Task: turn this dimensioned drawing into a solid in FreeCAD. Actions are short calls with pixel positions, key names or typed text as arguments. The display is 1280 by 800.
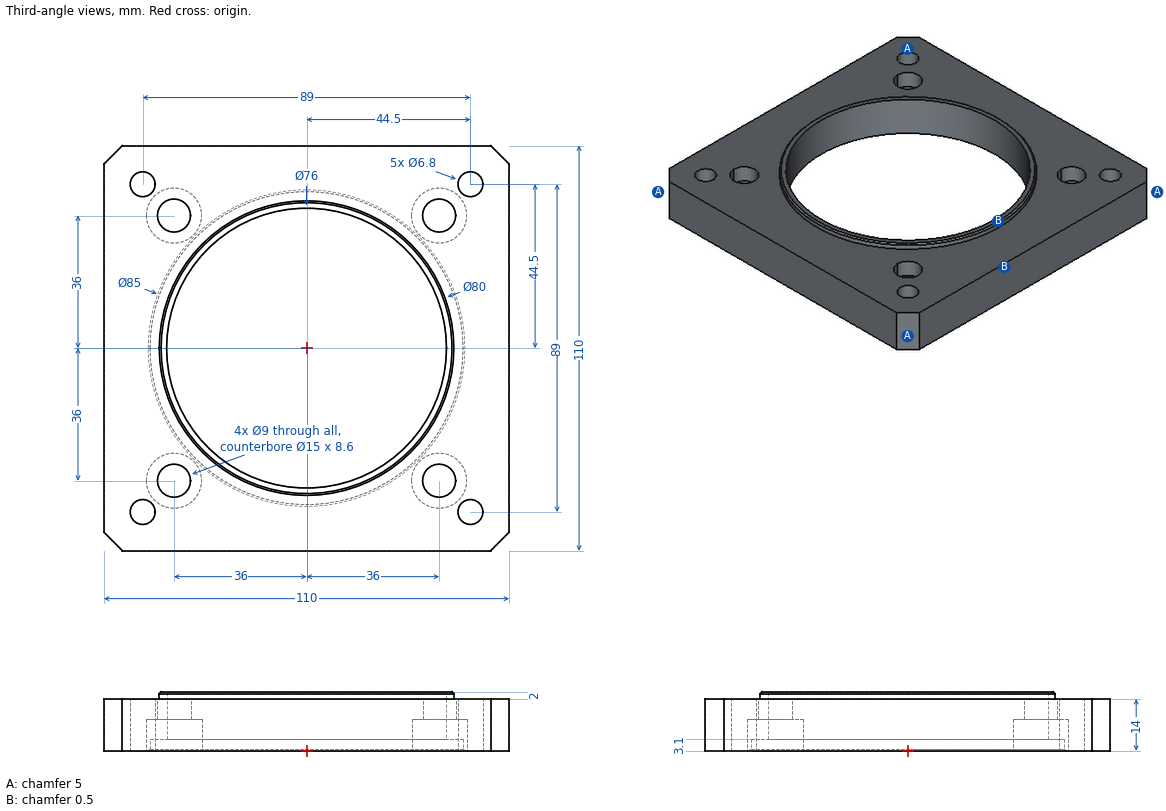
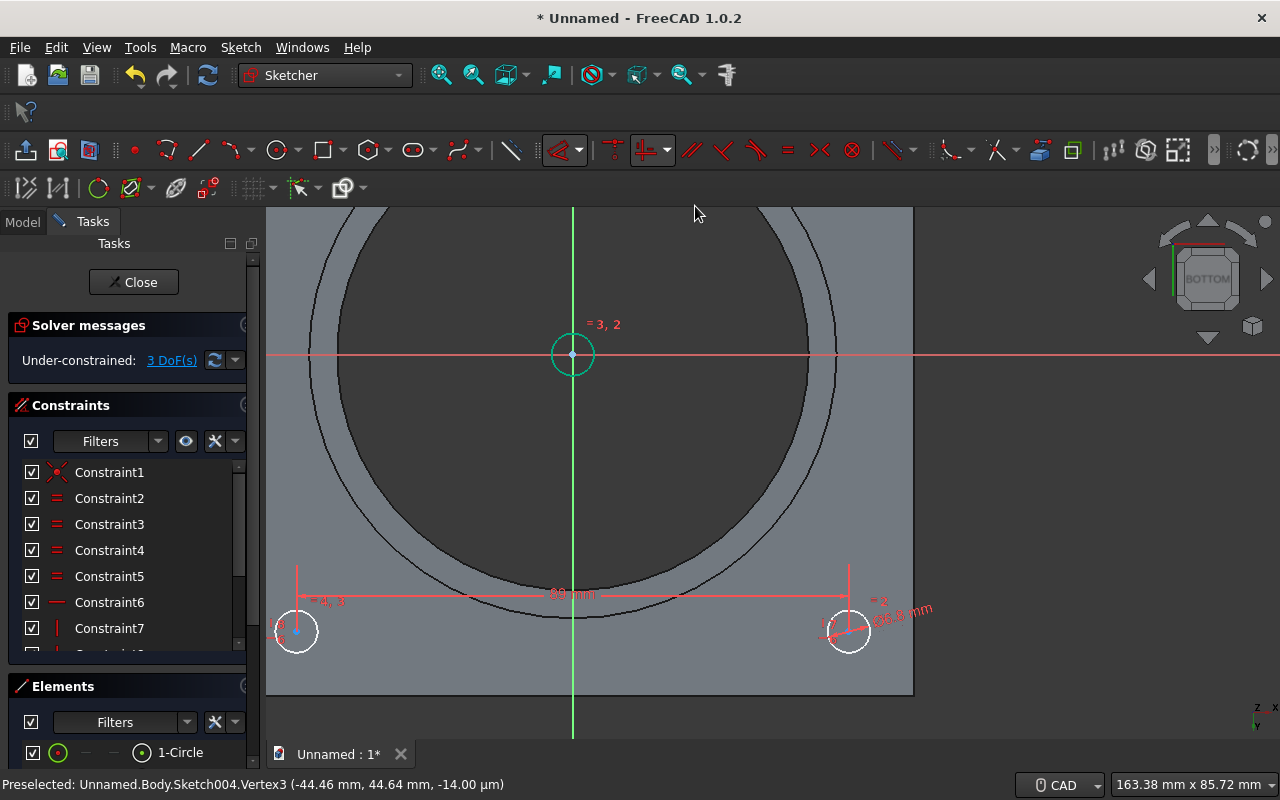
click(849, 632)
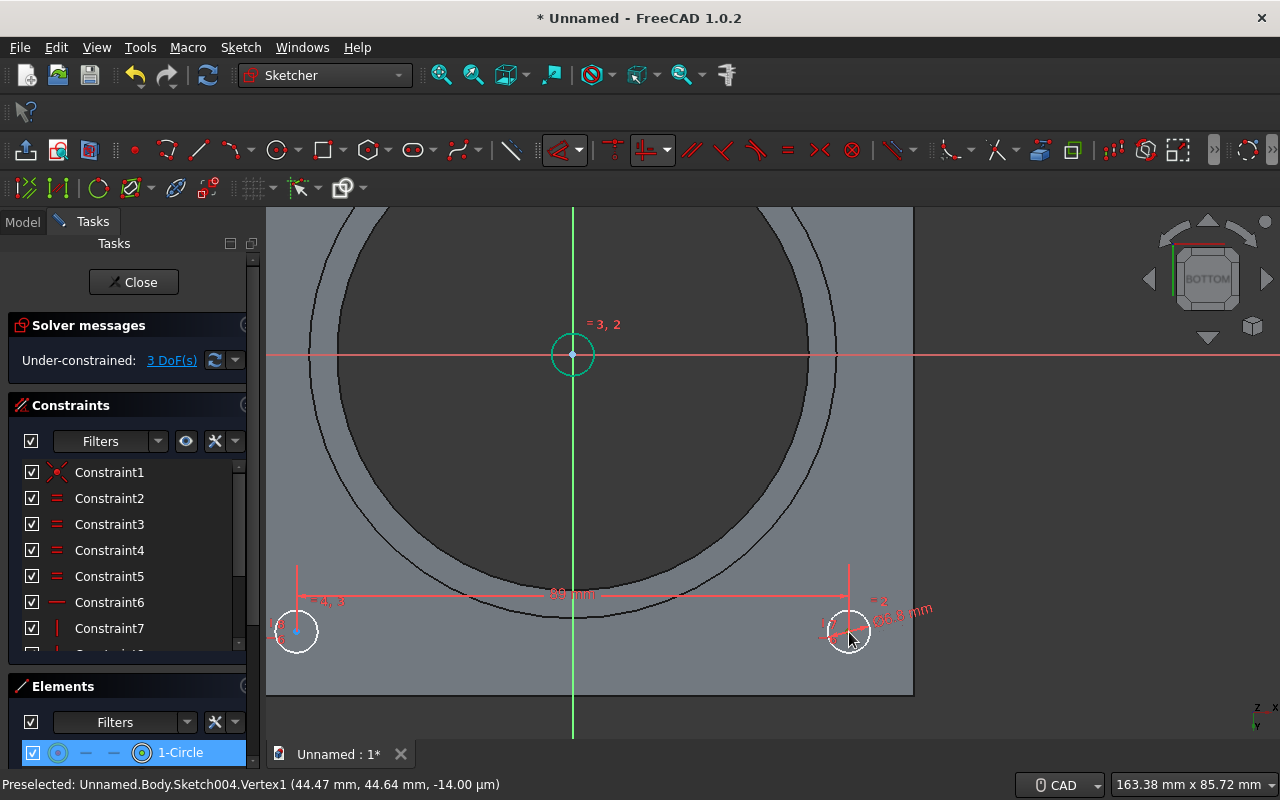
scroll(865, 617, down, 3)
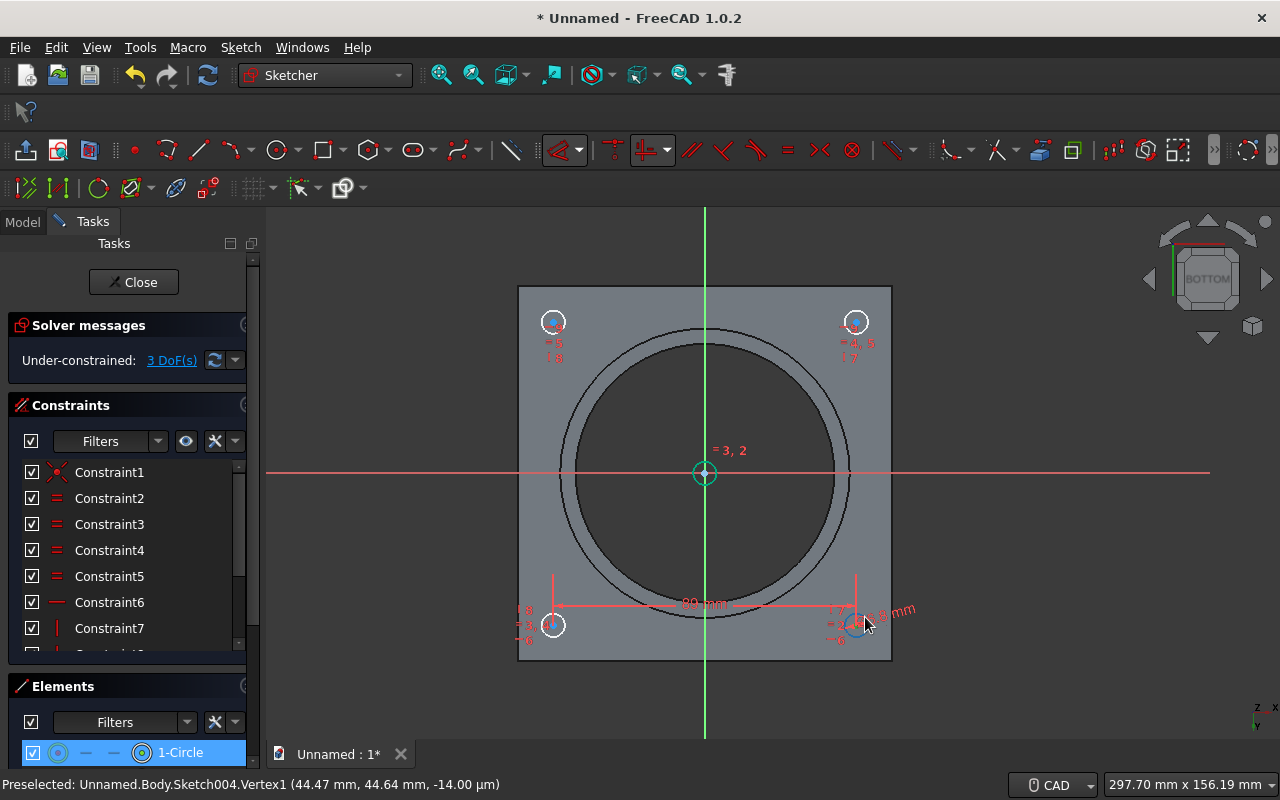
click(856, 322)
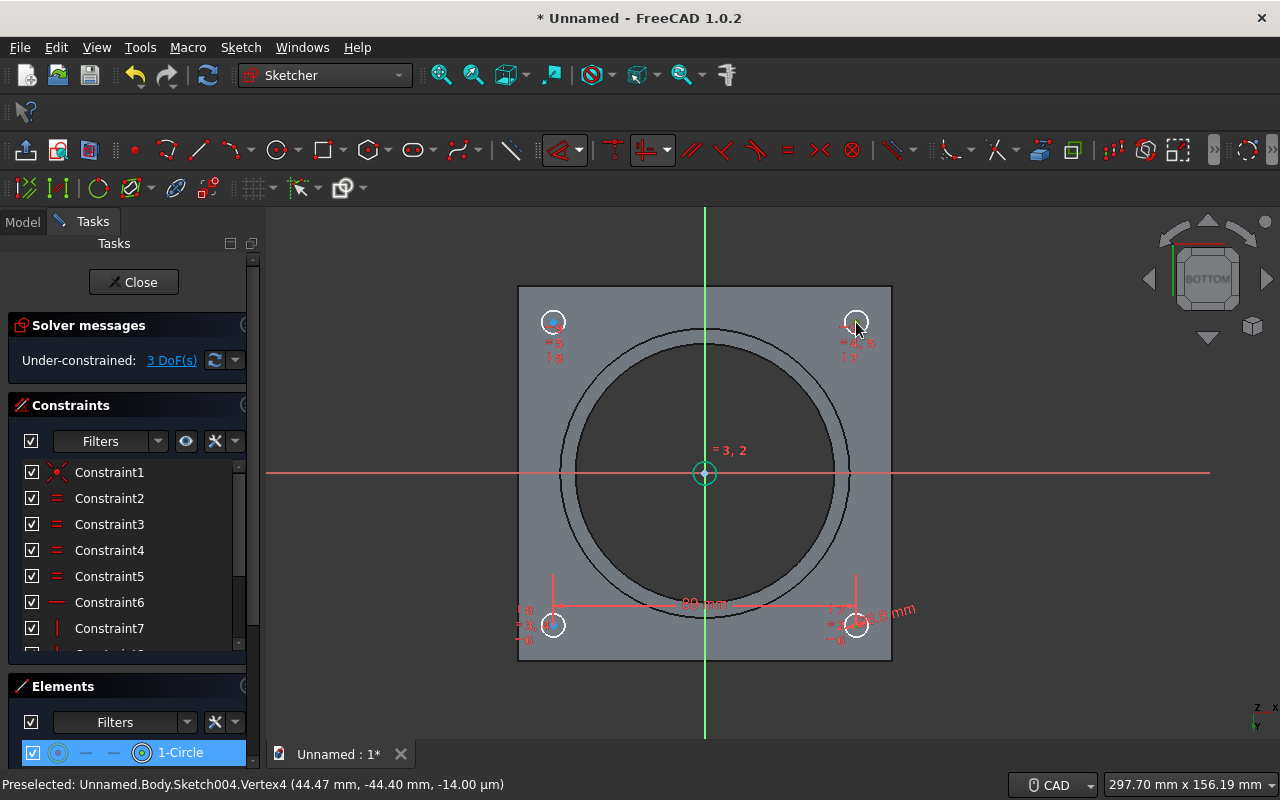
key(i)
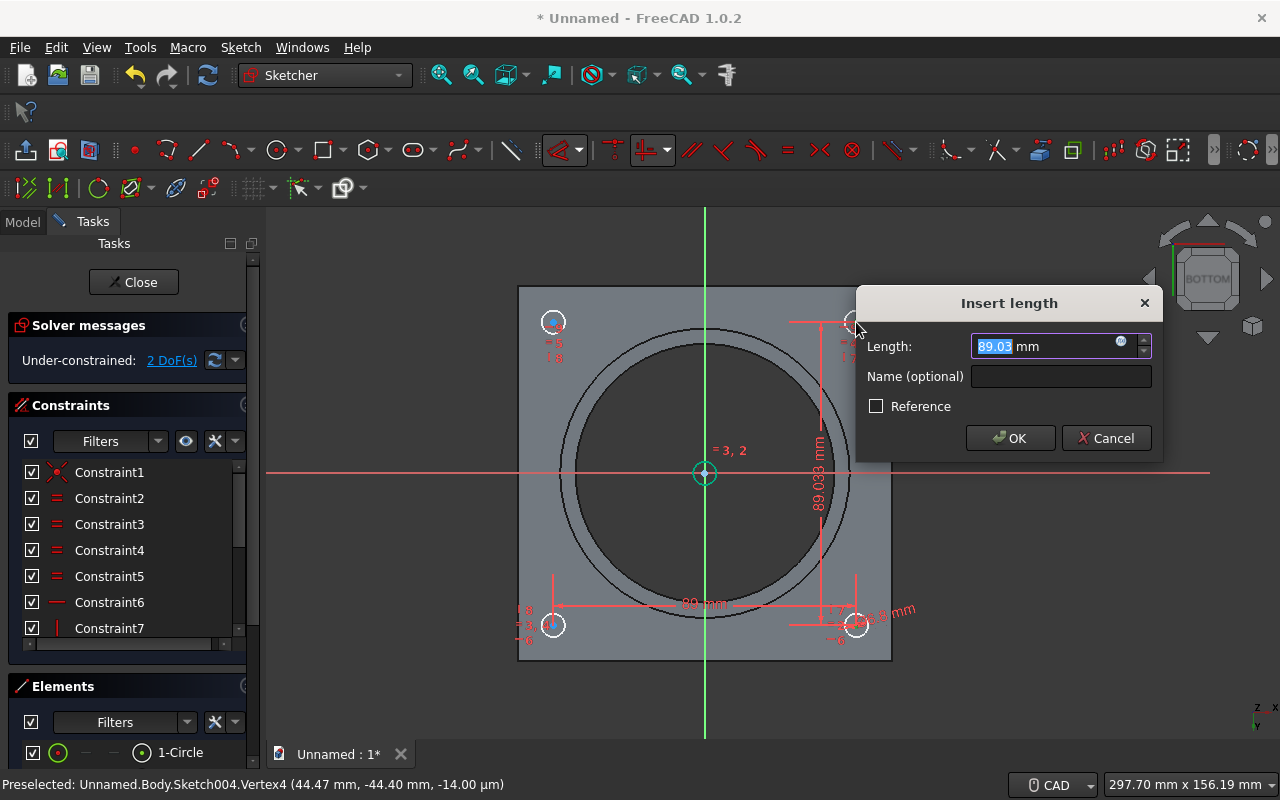
text(89)
key(Return)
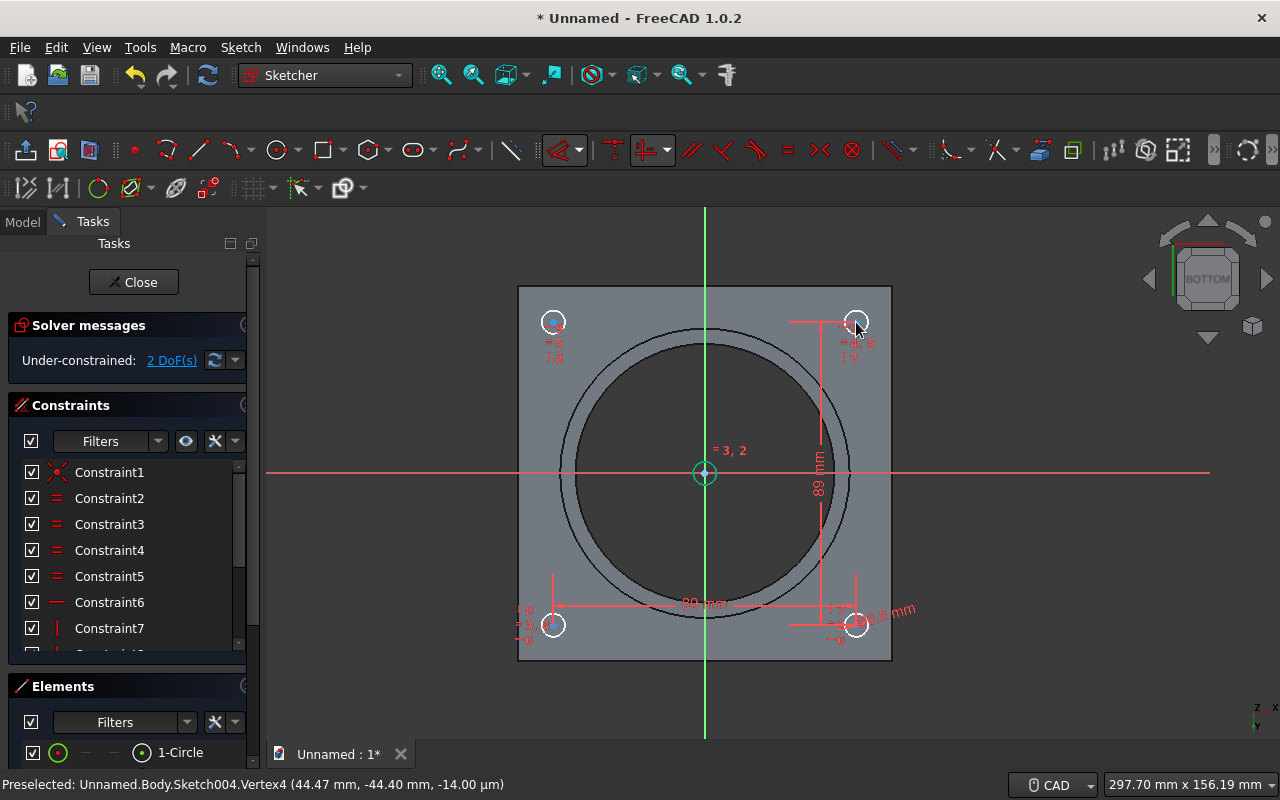
click(856, 625)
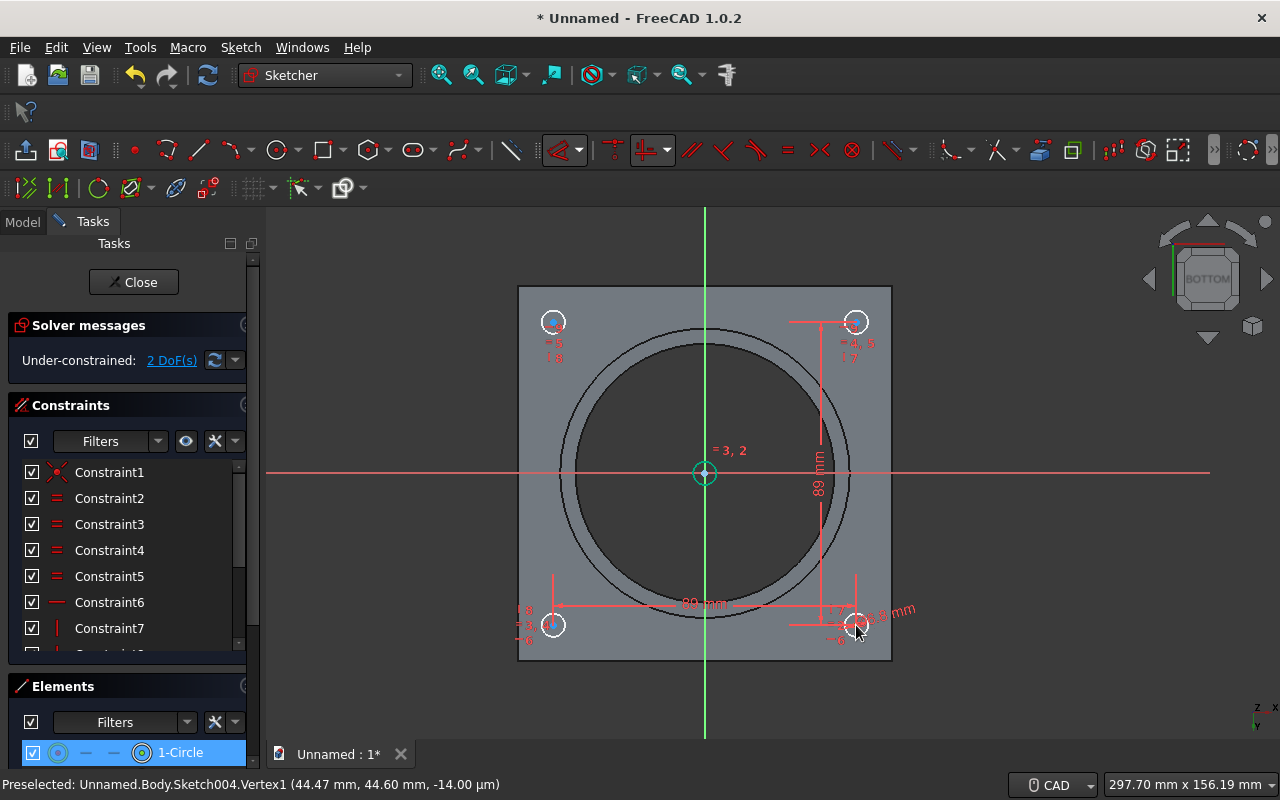
key(l)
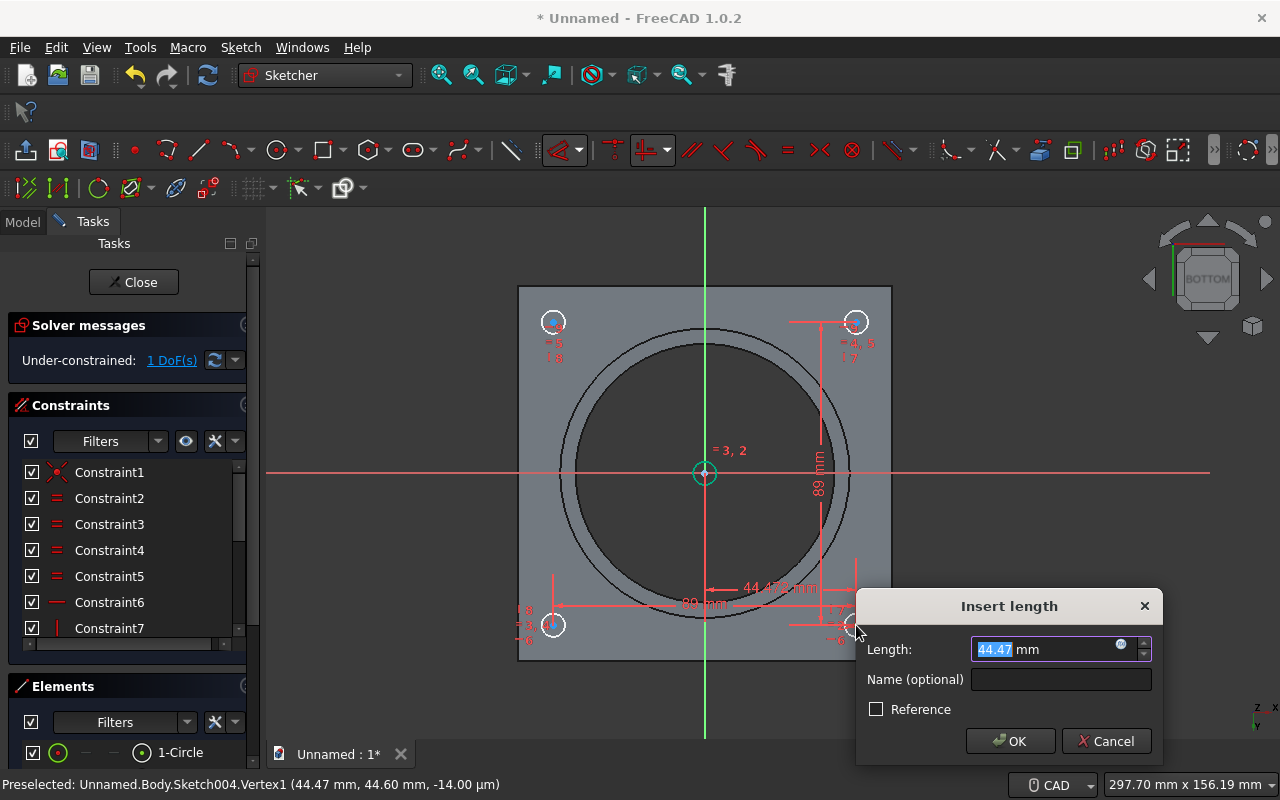
text(44.5)
key(Return)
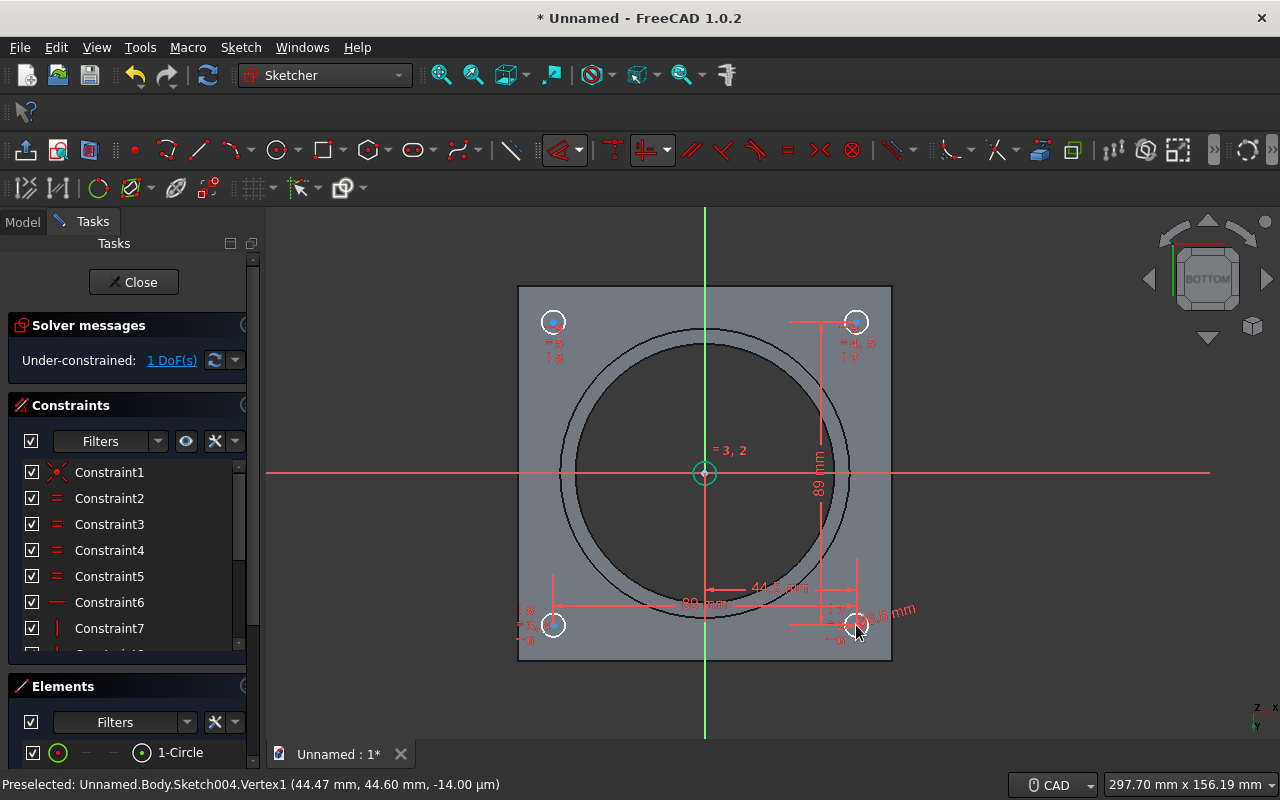
click(857, 625)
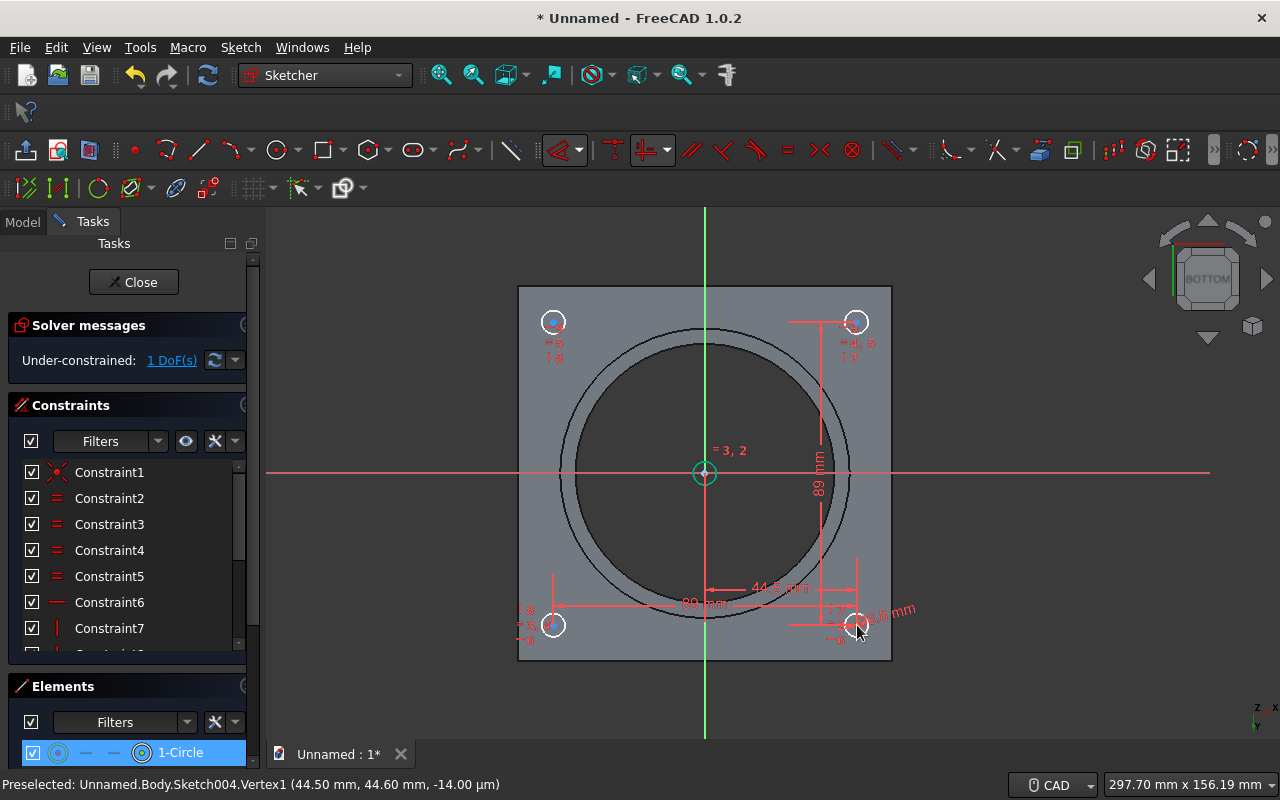
click(582, 150)